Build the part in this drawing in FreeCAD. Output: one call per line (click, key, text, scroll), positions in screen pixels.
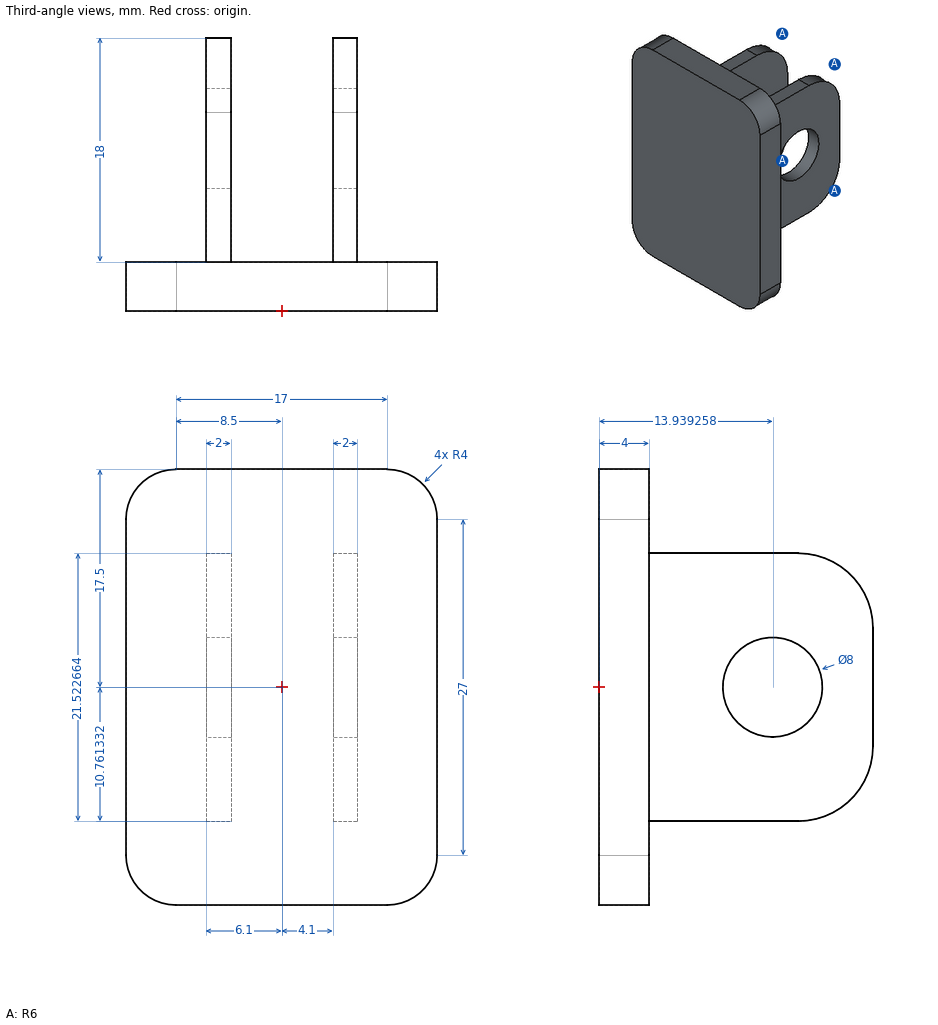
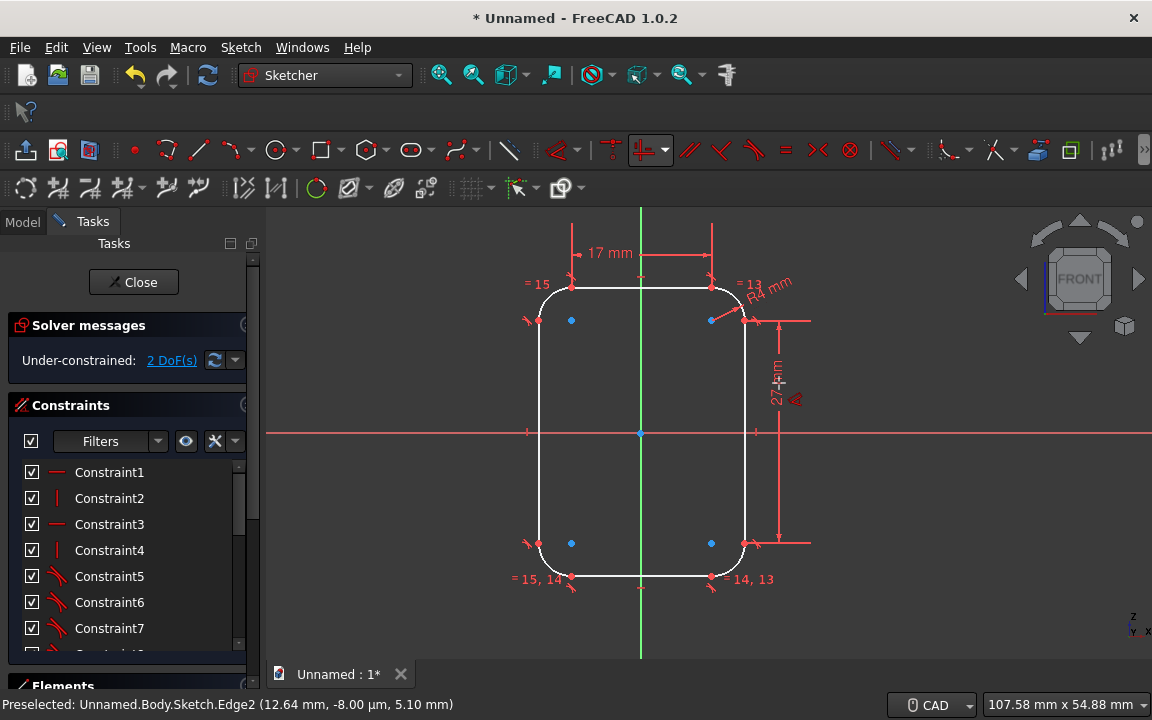
click(572, 288)
click(606, 467)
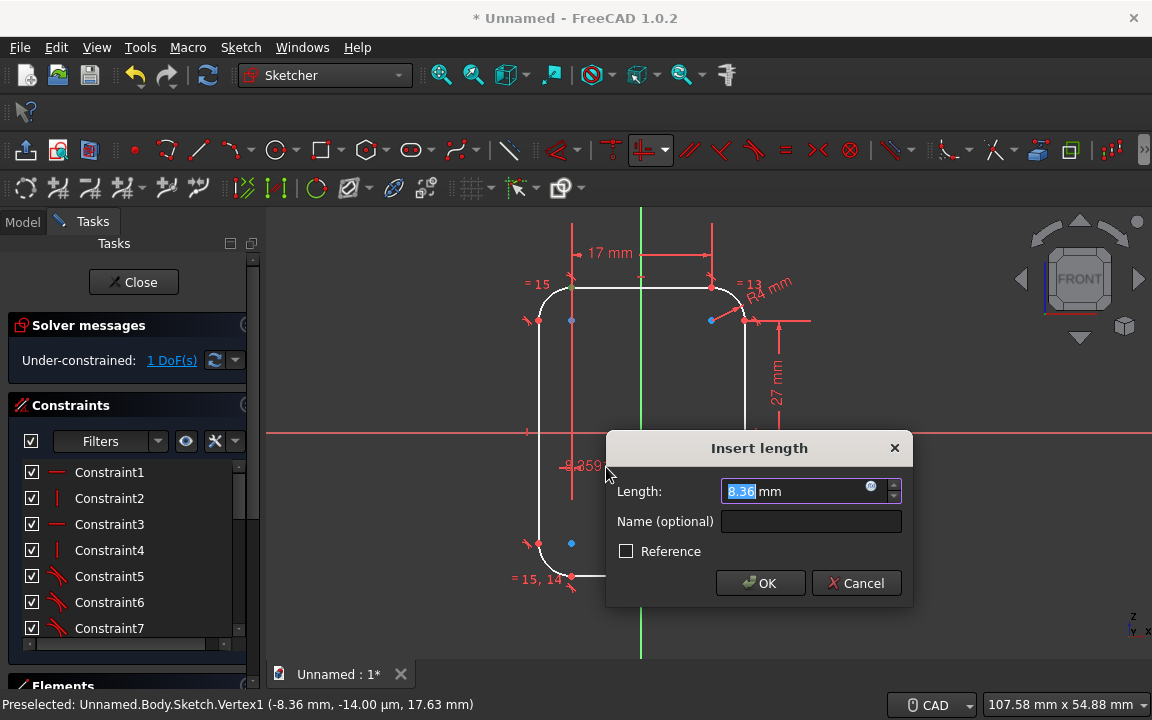
text(8.5)
key(Return)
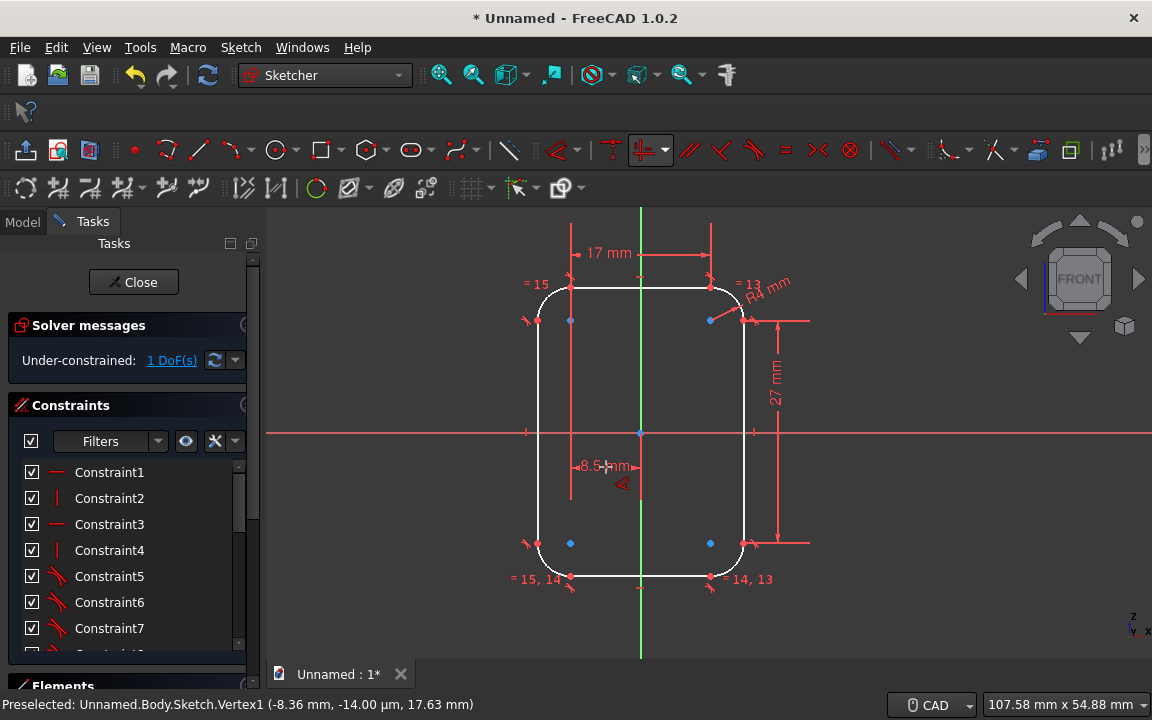
click(571, 288)
click(675, 360)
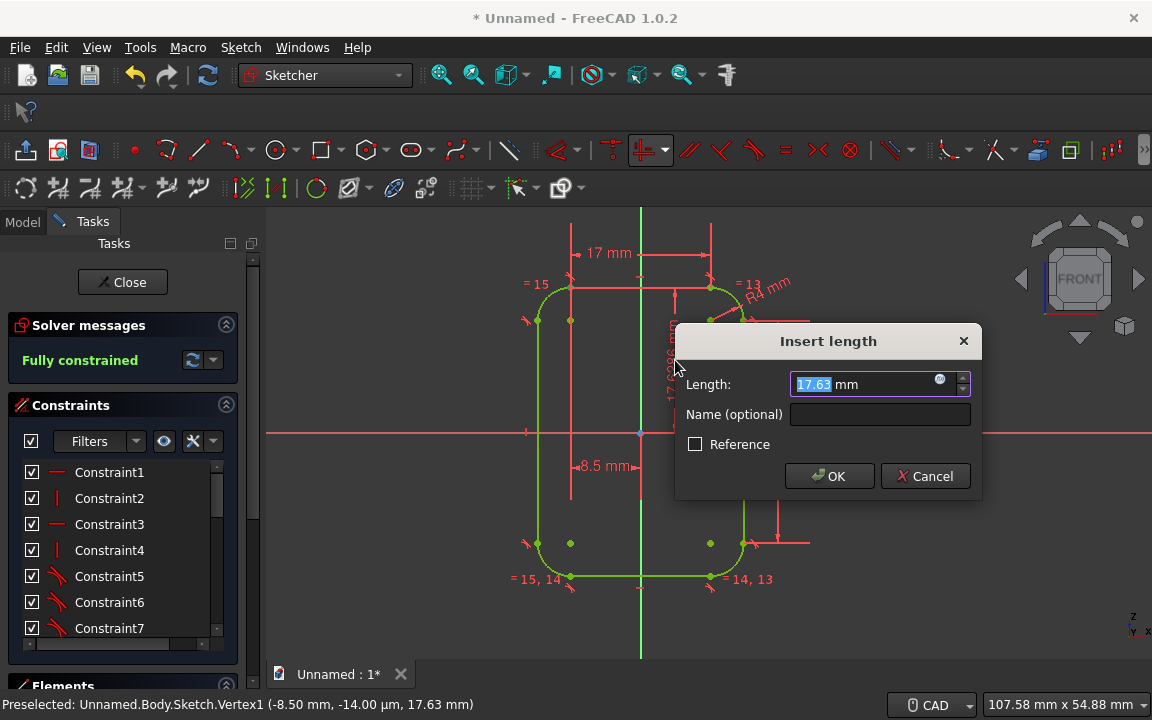
text(17.5)
key(Return)
key(Escape)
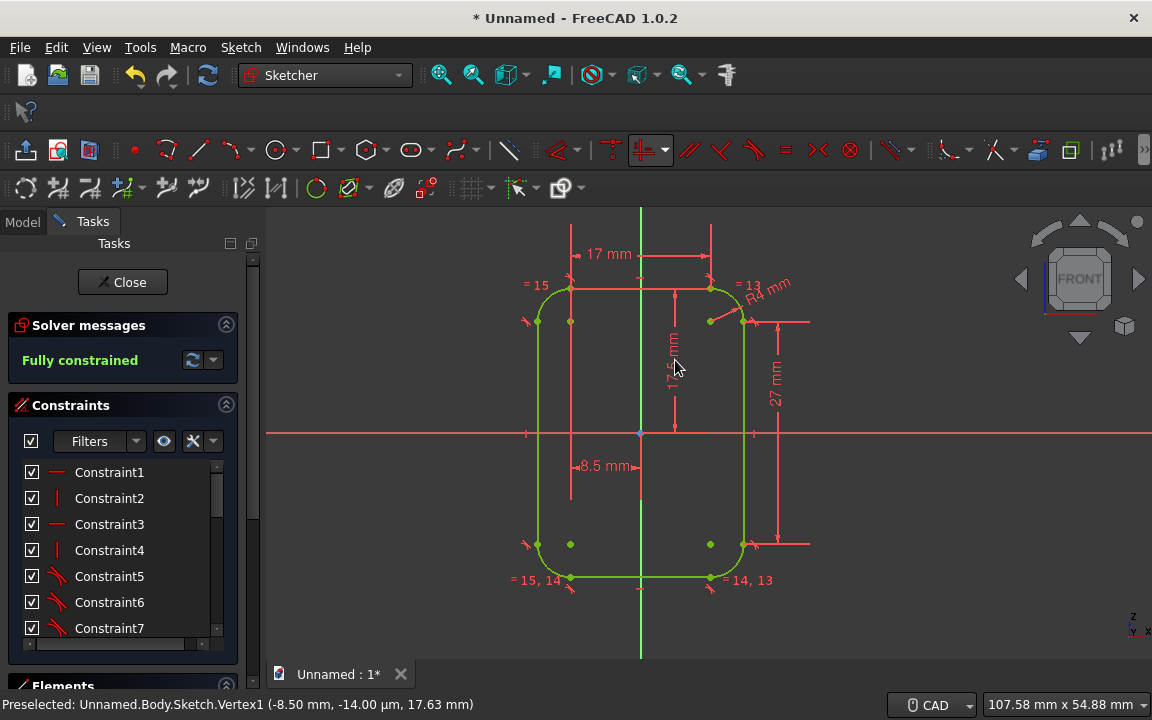
click(123, 282)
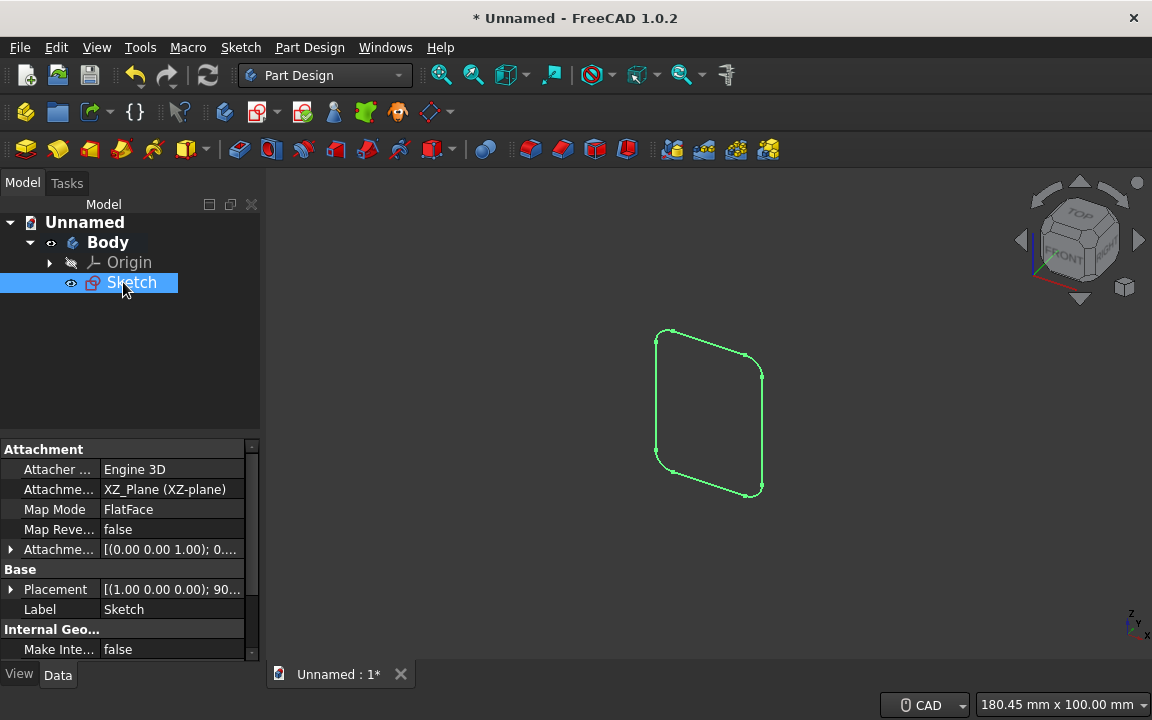
click(26, 150)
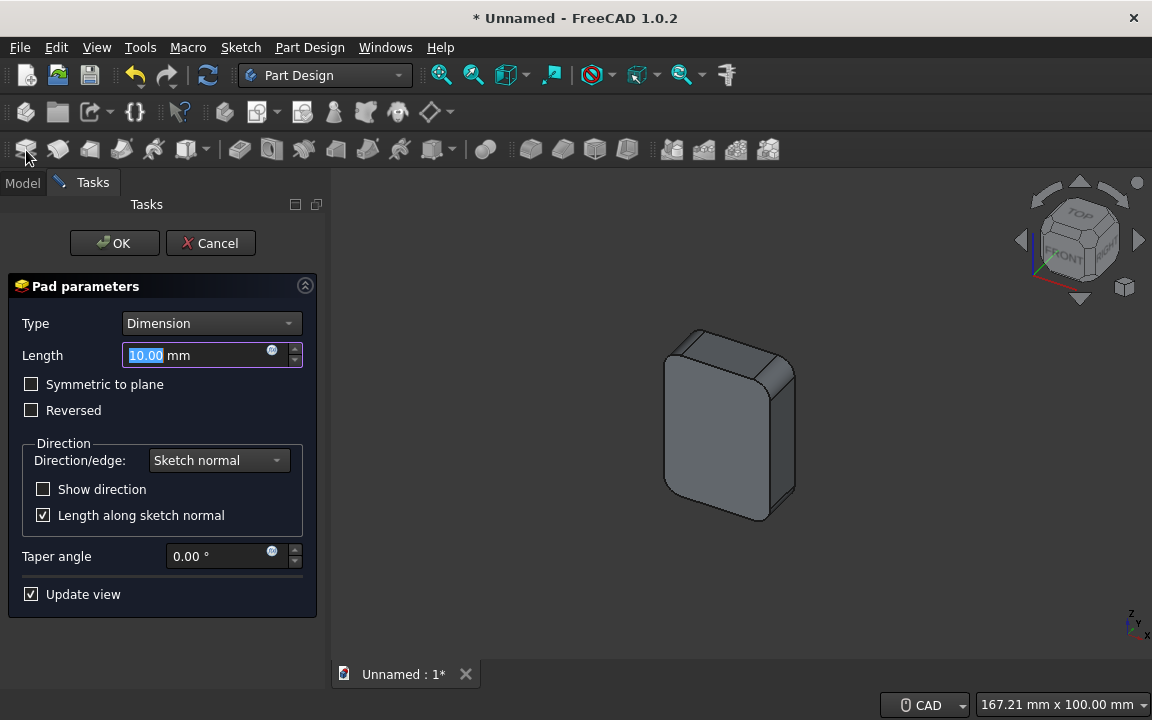
text(4)
key(Tab)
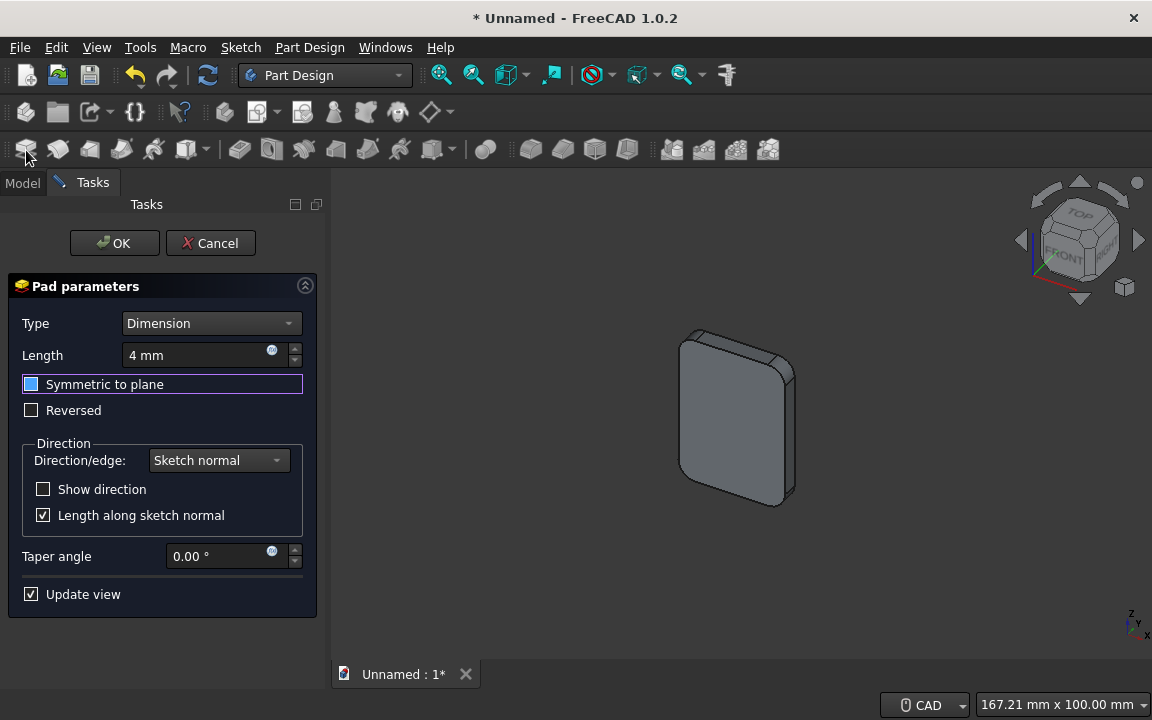
click(30, 410)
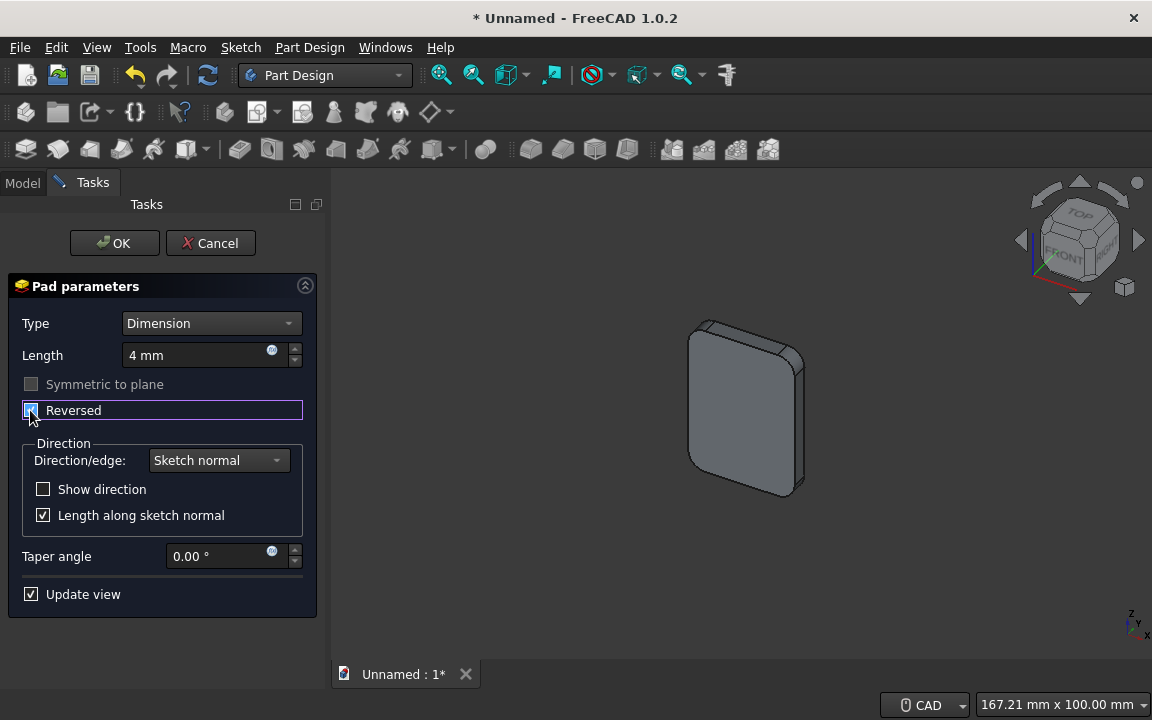
click(115, 243)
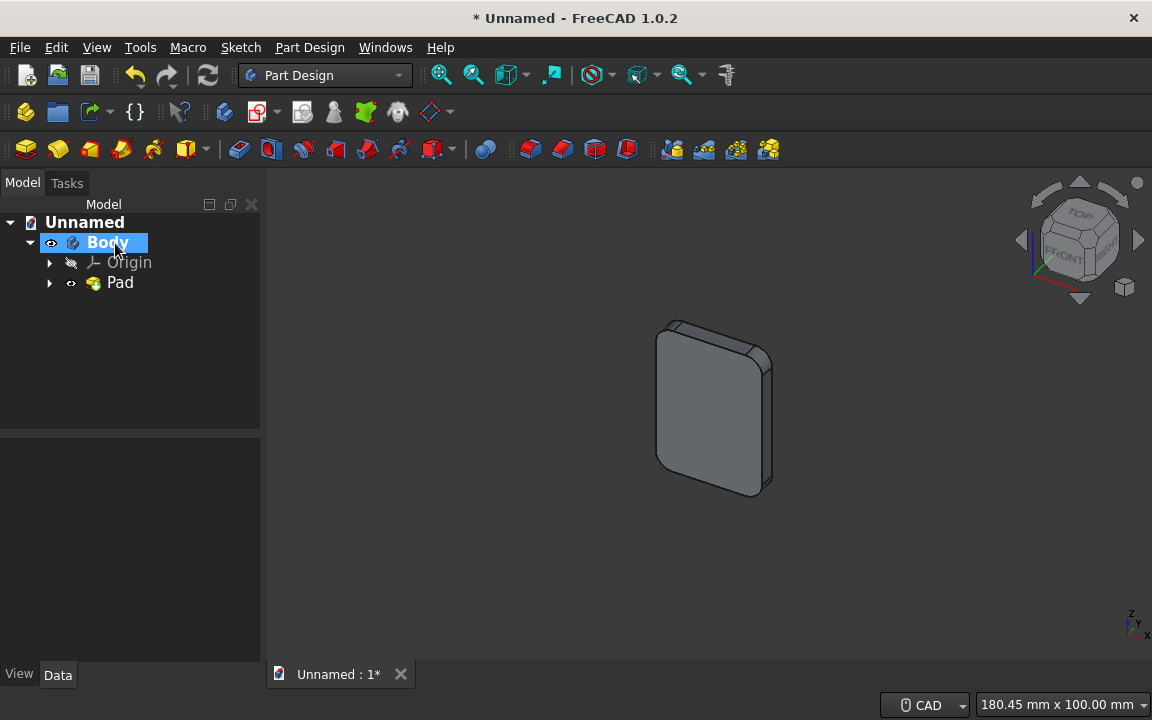
click(442, 76)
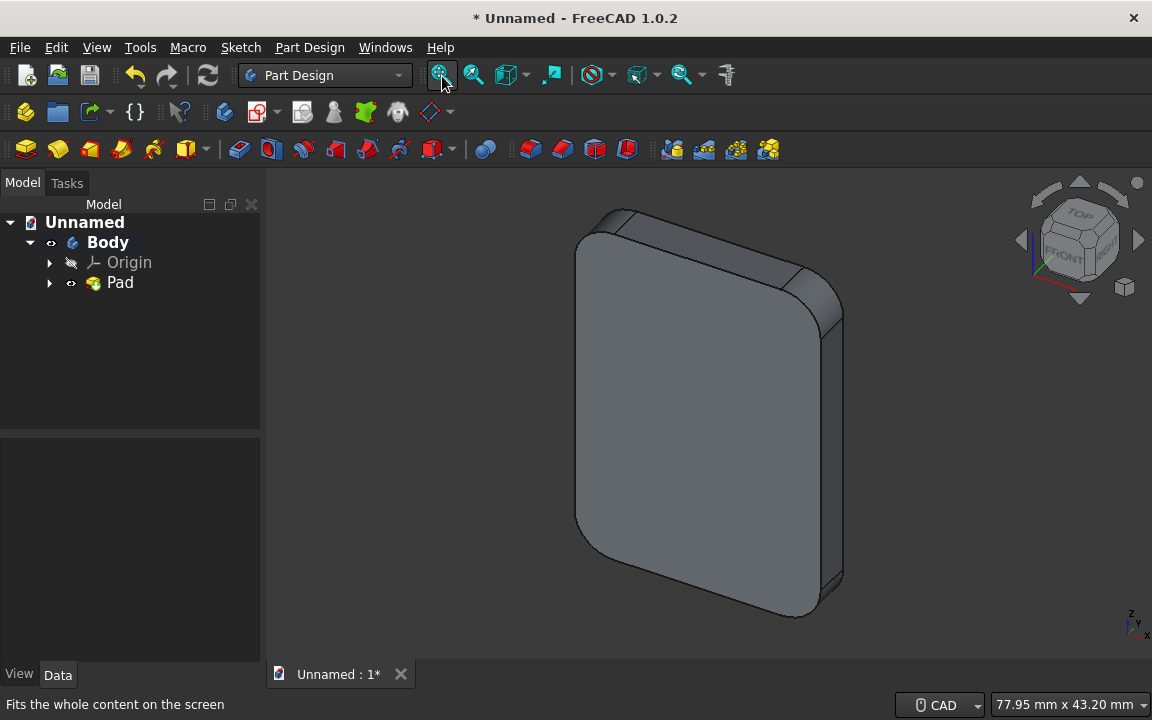
key(4)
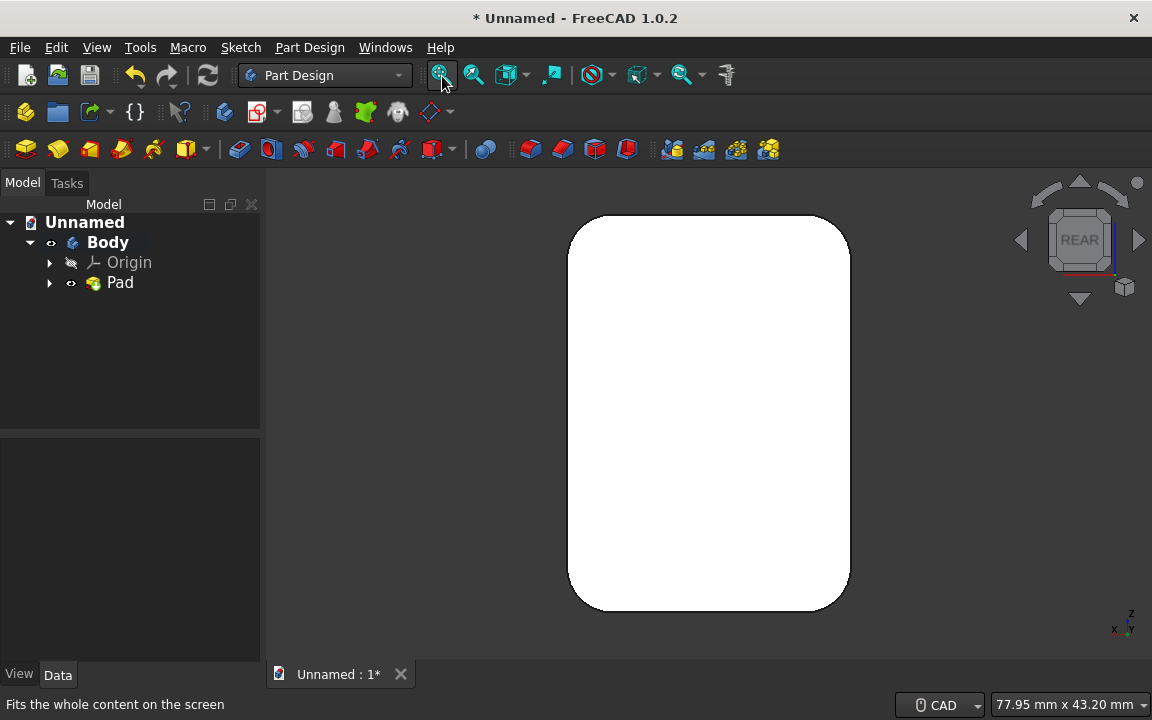
click(709, 356)